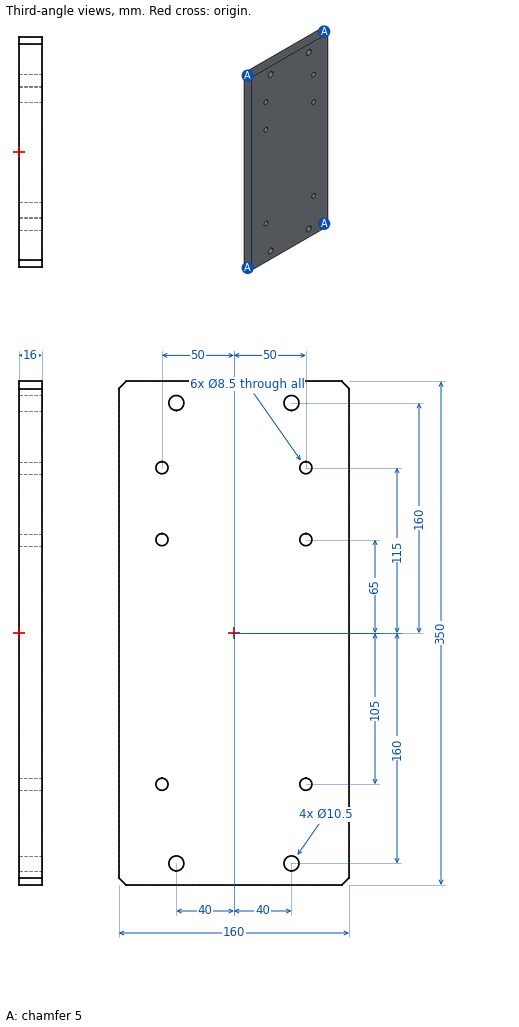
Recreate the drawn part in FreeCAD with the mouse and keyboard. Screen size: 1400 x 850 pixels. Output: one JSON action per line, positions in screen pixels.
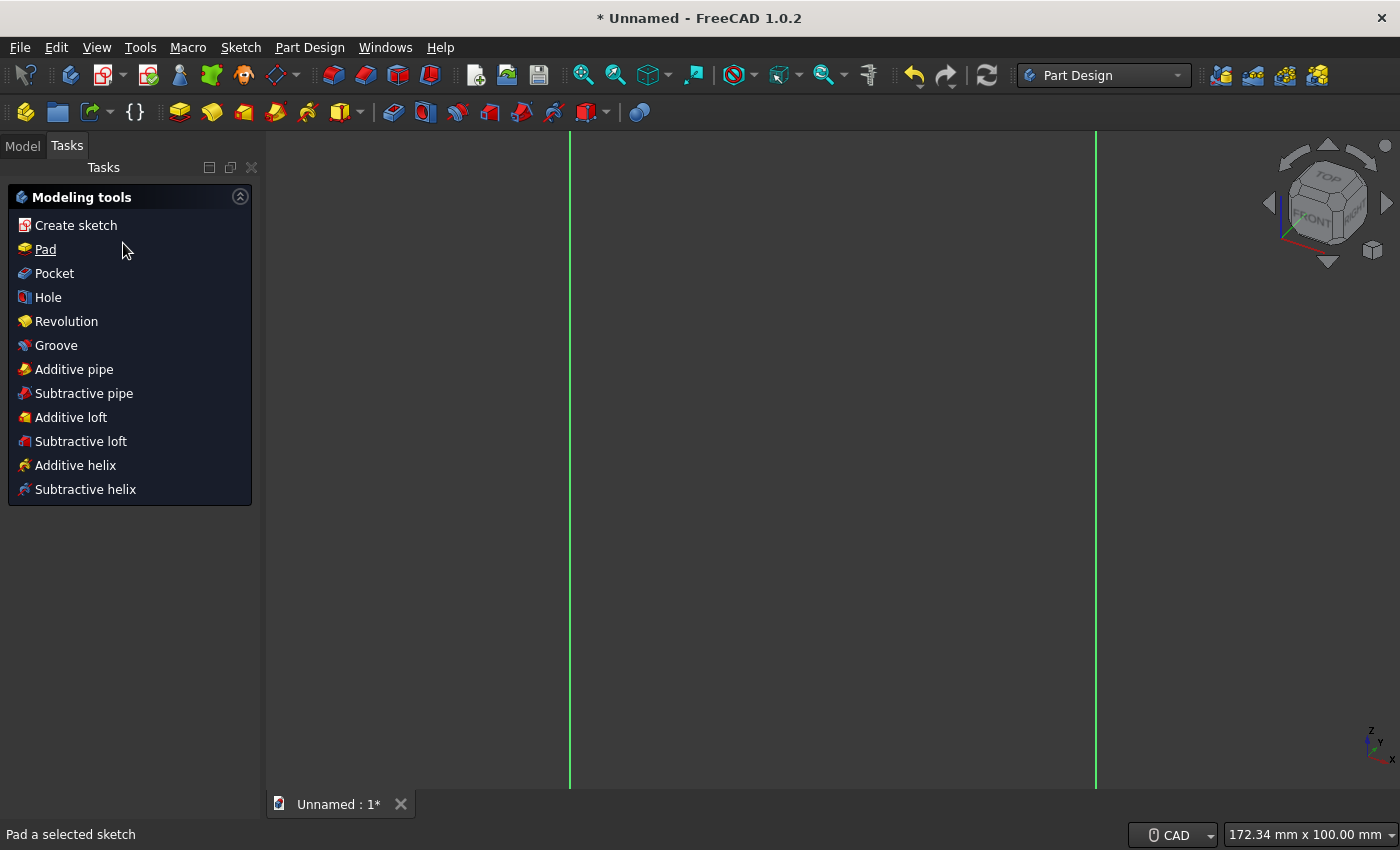
{"action": "left_click", "coordinate": [180, 112]}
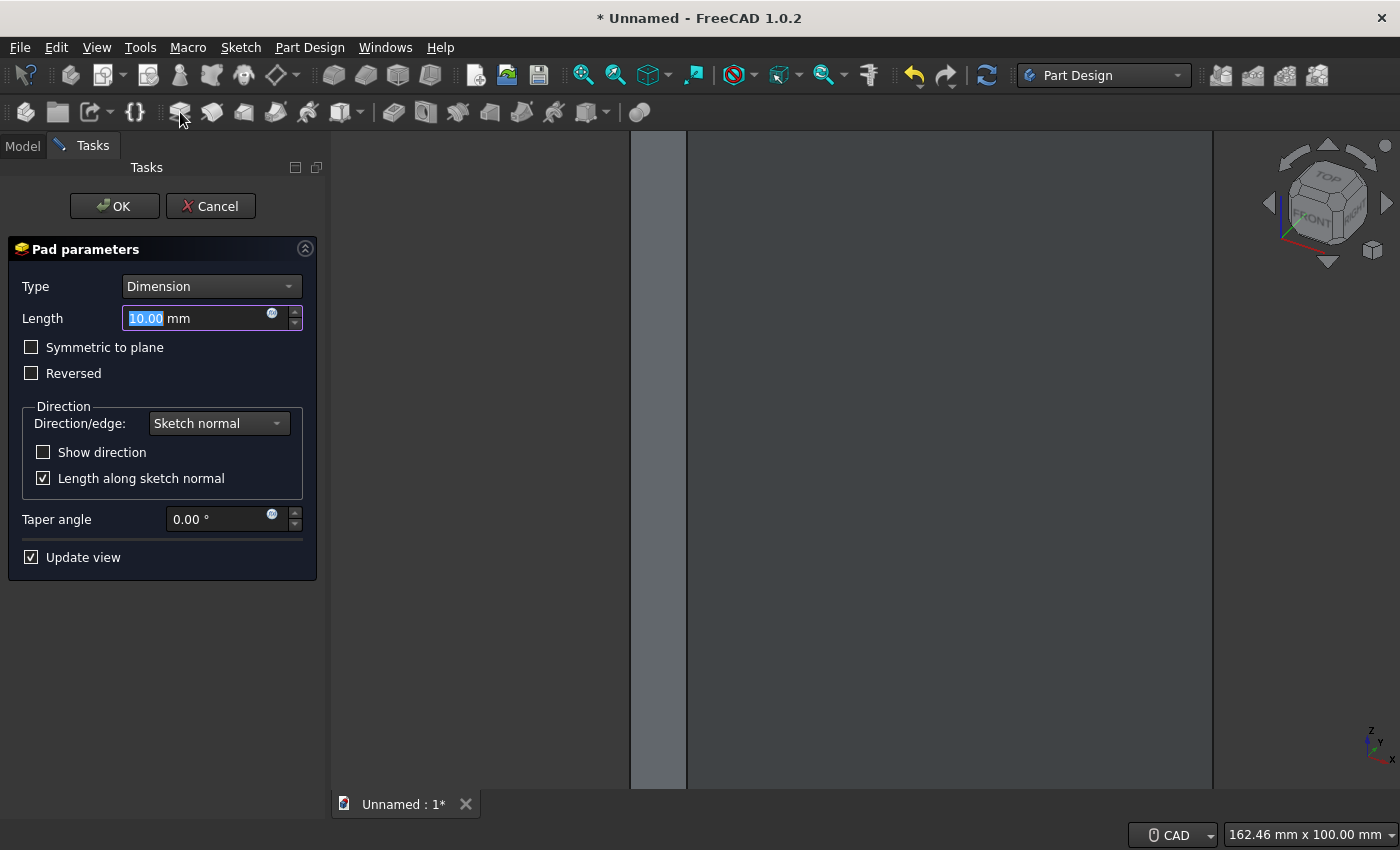
{"action": "type", "text": "16"}
{"action": "key", "text": "Tab"}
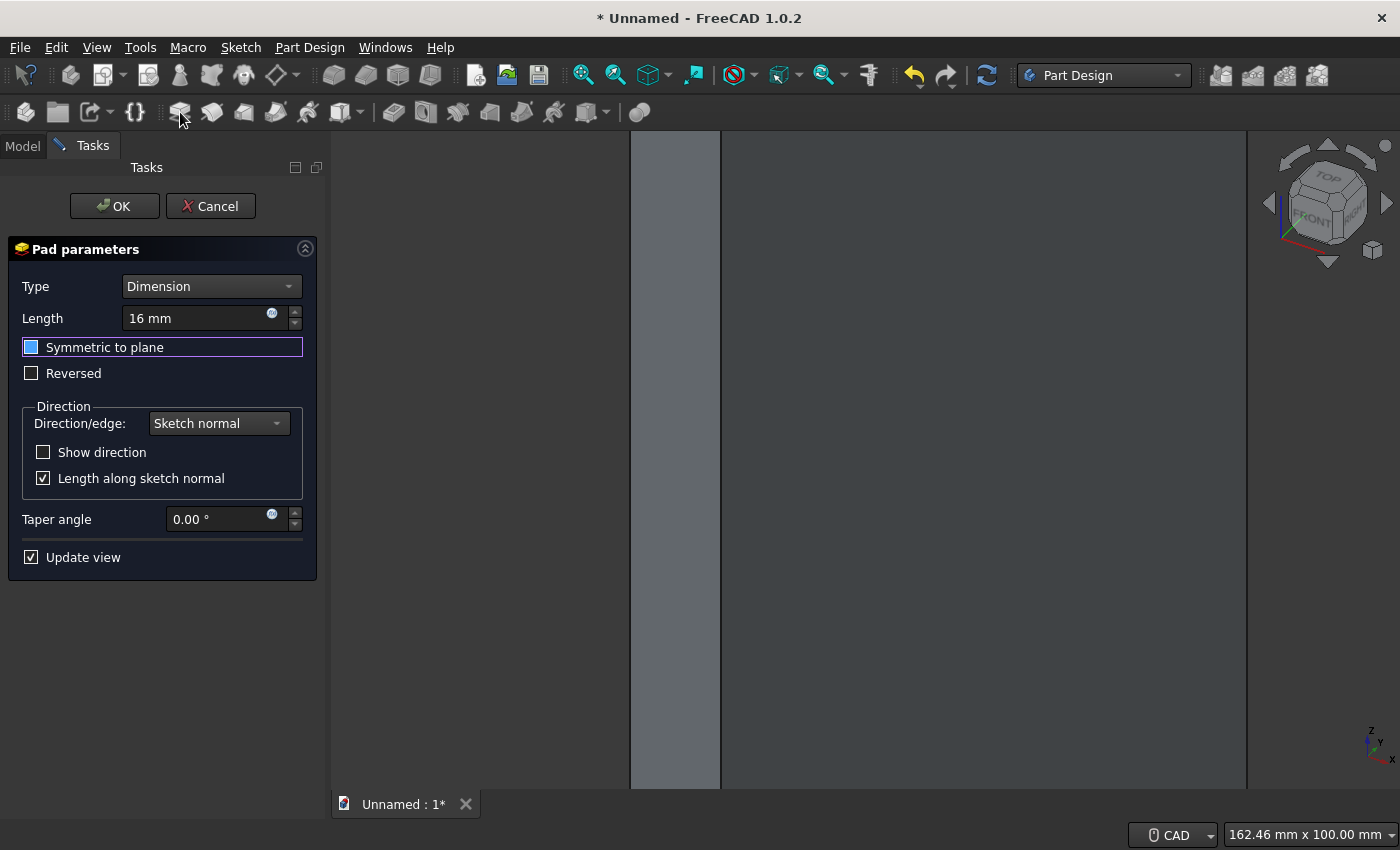
{"action": "left_click", "coordinate": [115, 206]}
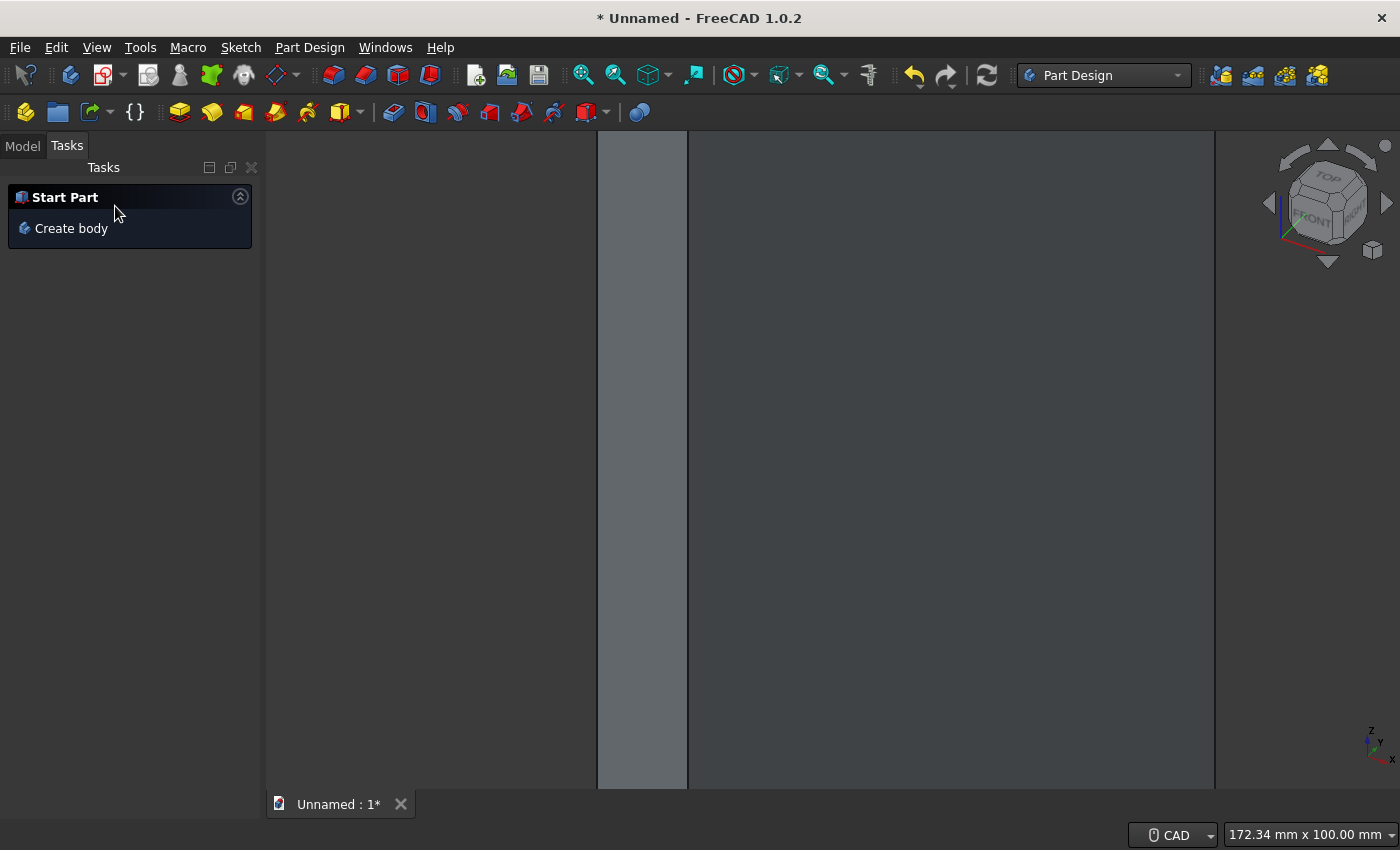
{"action": "key", "text": "v f"}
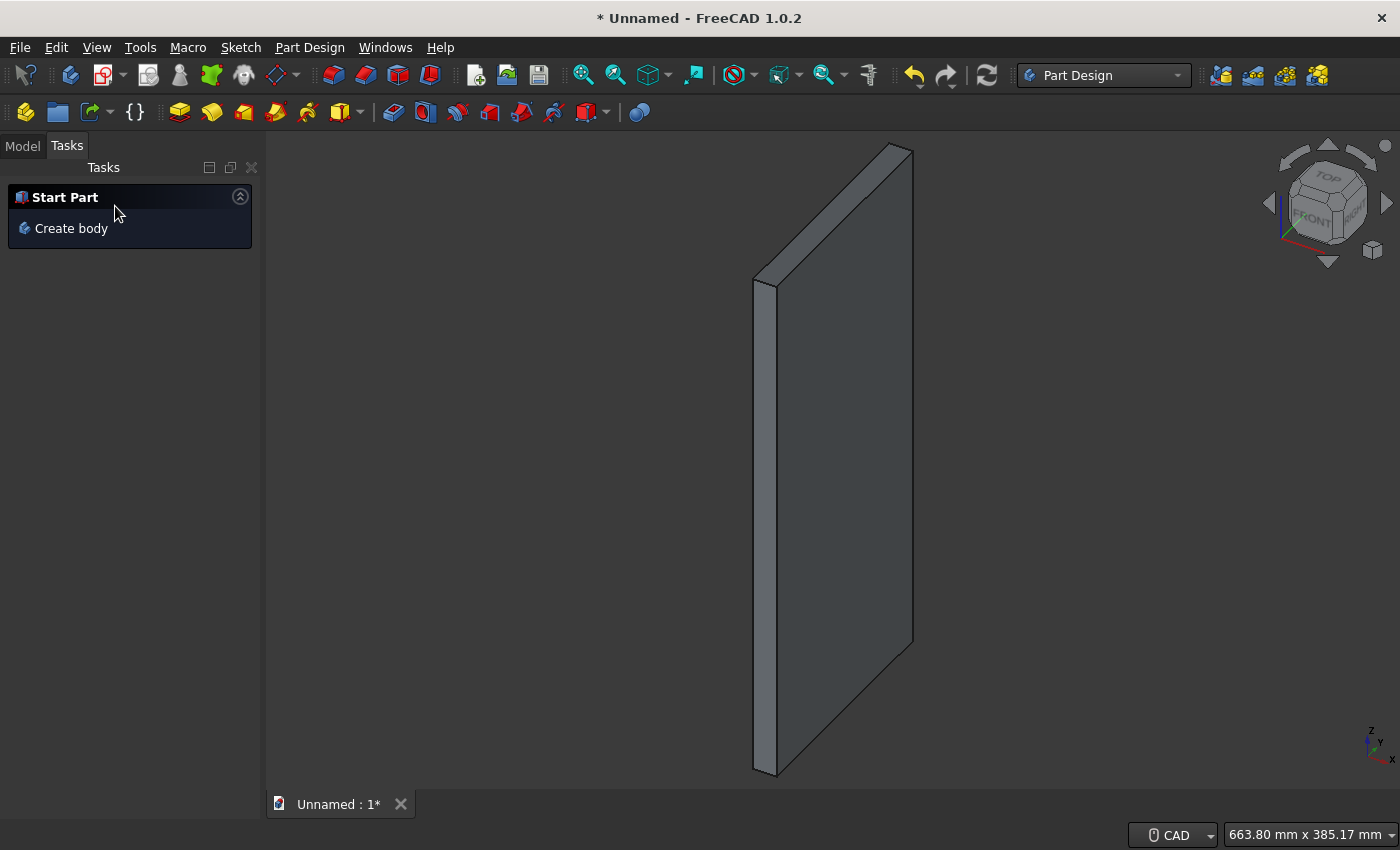
{"action": "left_click", "coordinate": [845, 533]}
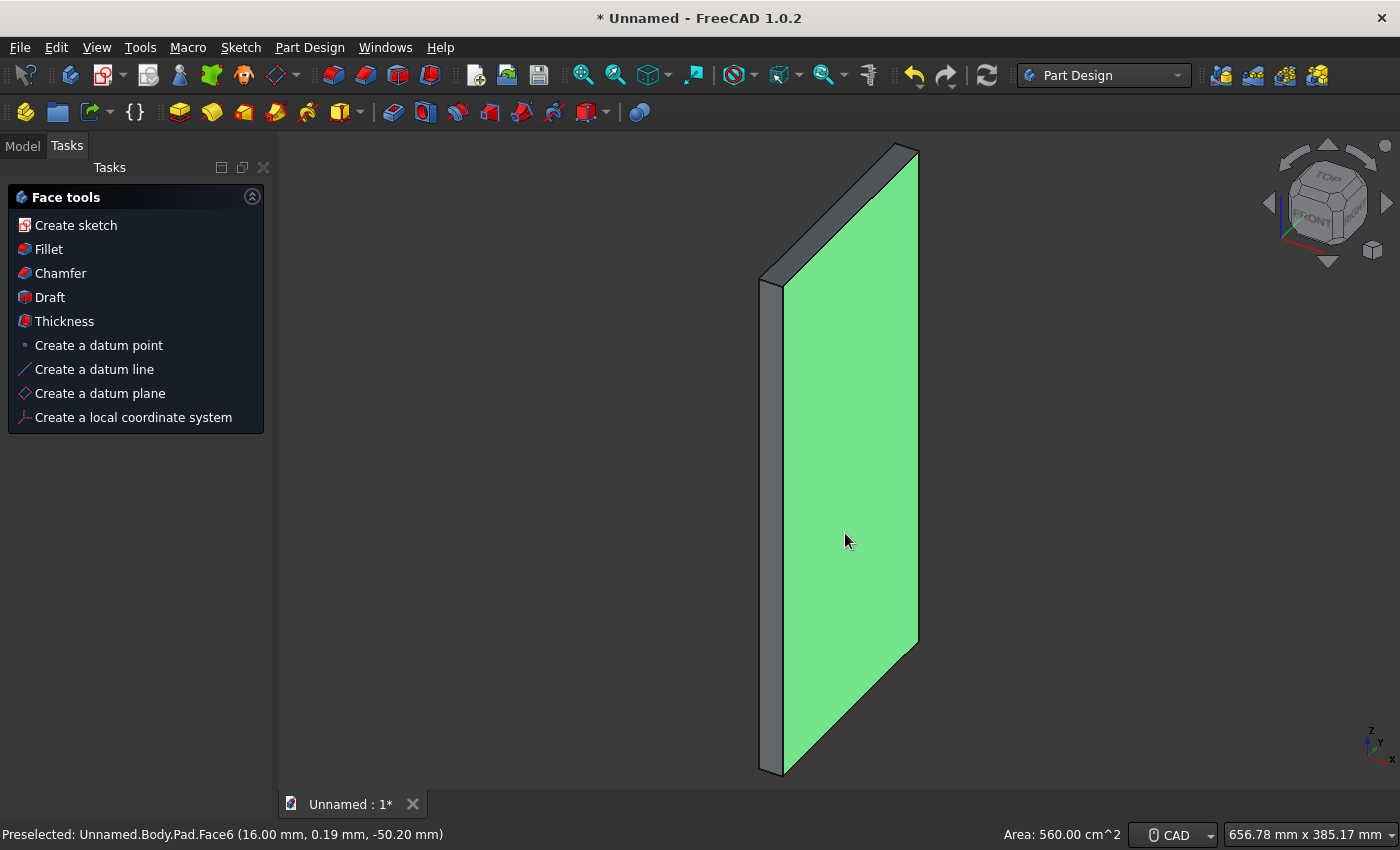
{"action": "left_click", "coordinate": [104, 76]}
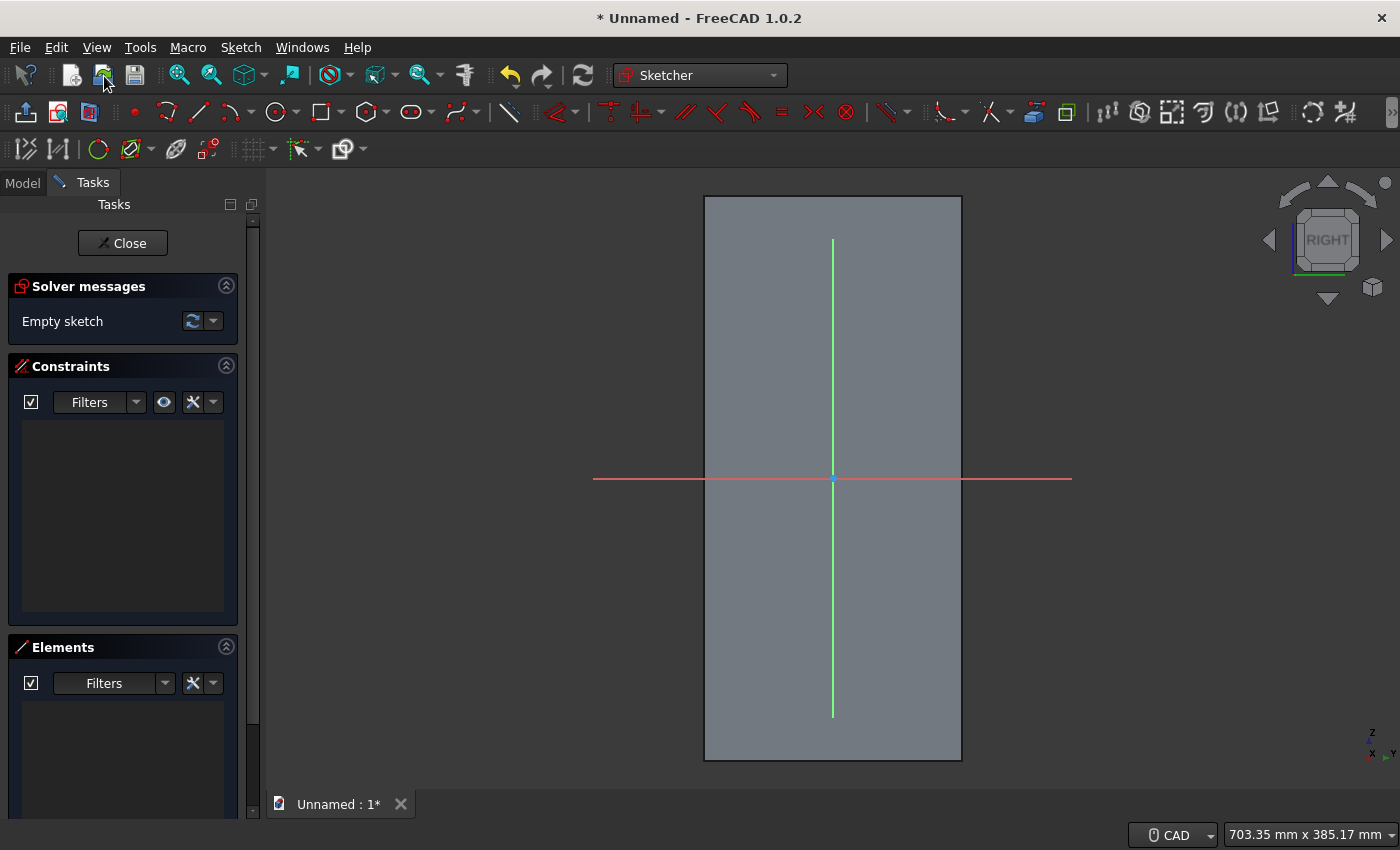
{"action": "key", "text": "g c"}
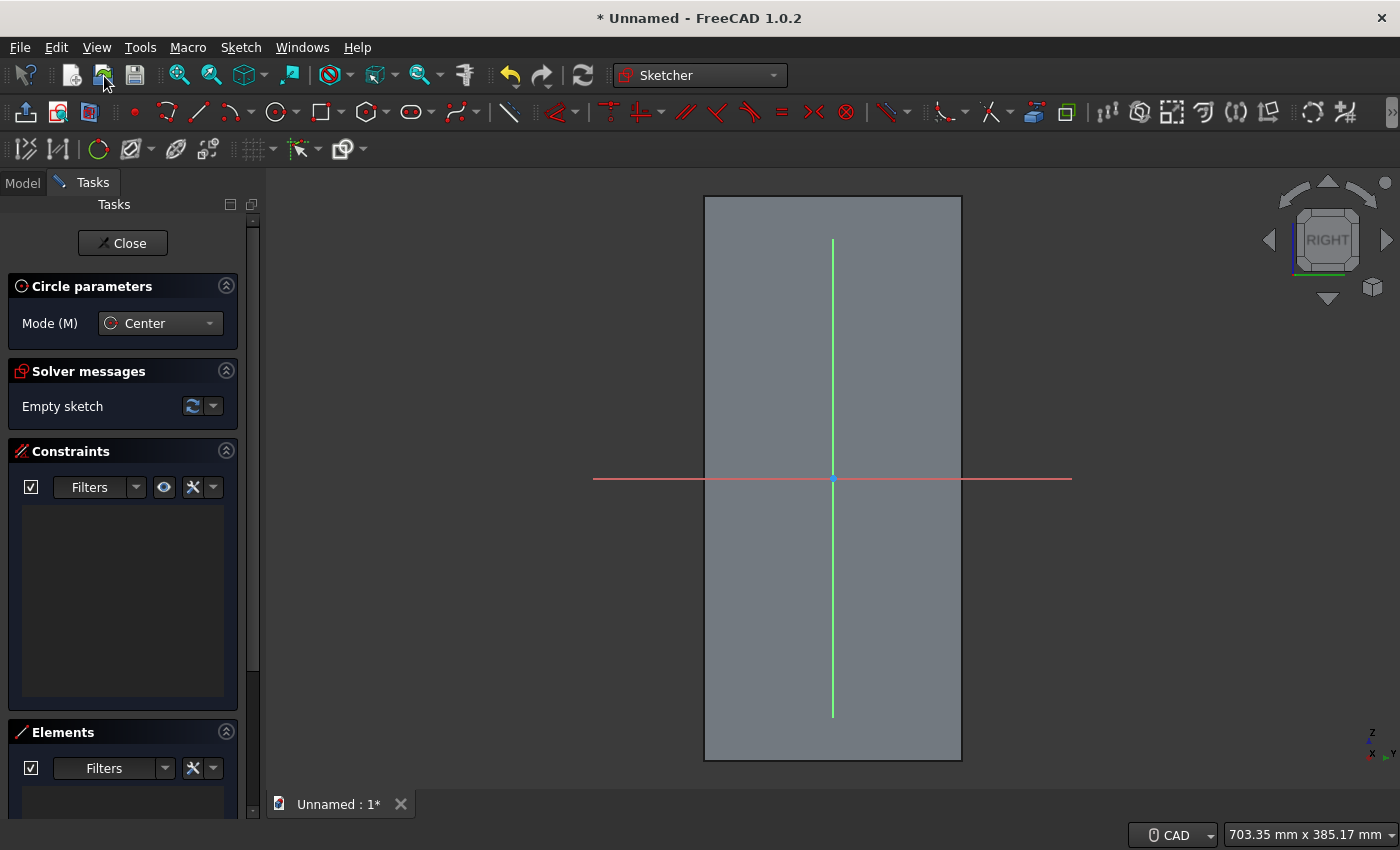
{"action": "scroll", "coordinate": [914, 293], "scroll_direction": "up", "scroll_amount": 6}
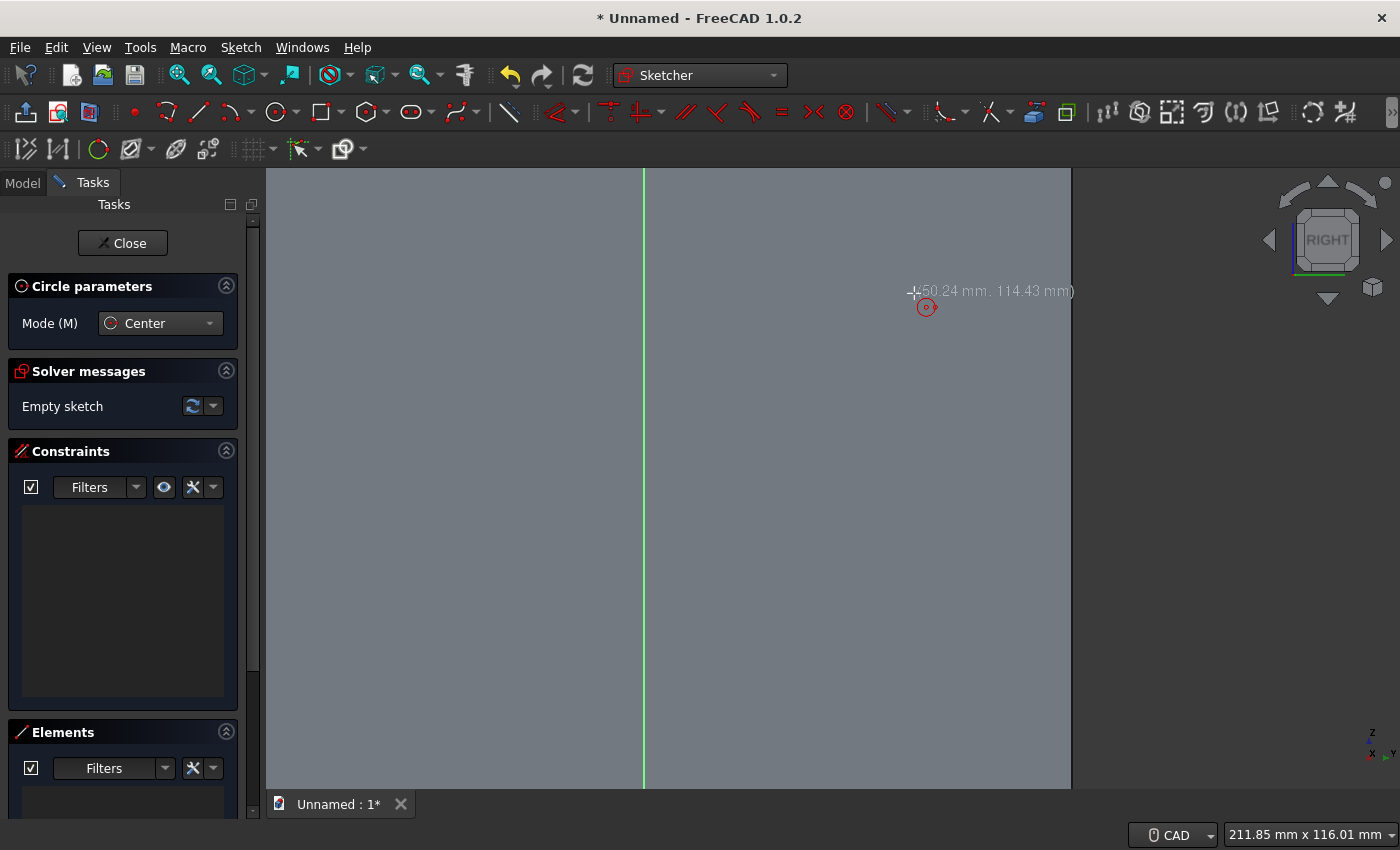
{"action": "left_click", "coordinate": [911, 293]}
{"action": "mouse_move", "coordinate": [927, 277]}